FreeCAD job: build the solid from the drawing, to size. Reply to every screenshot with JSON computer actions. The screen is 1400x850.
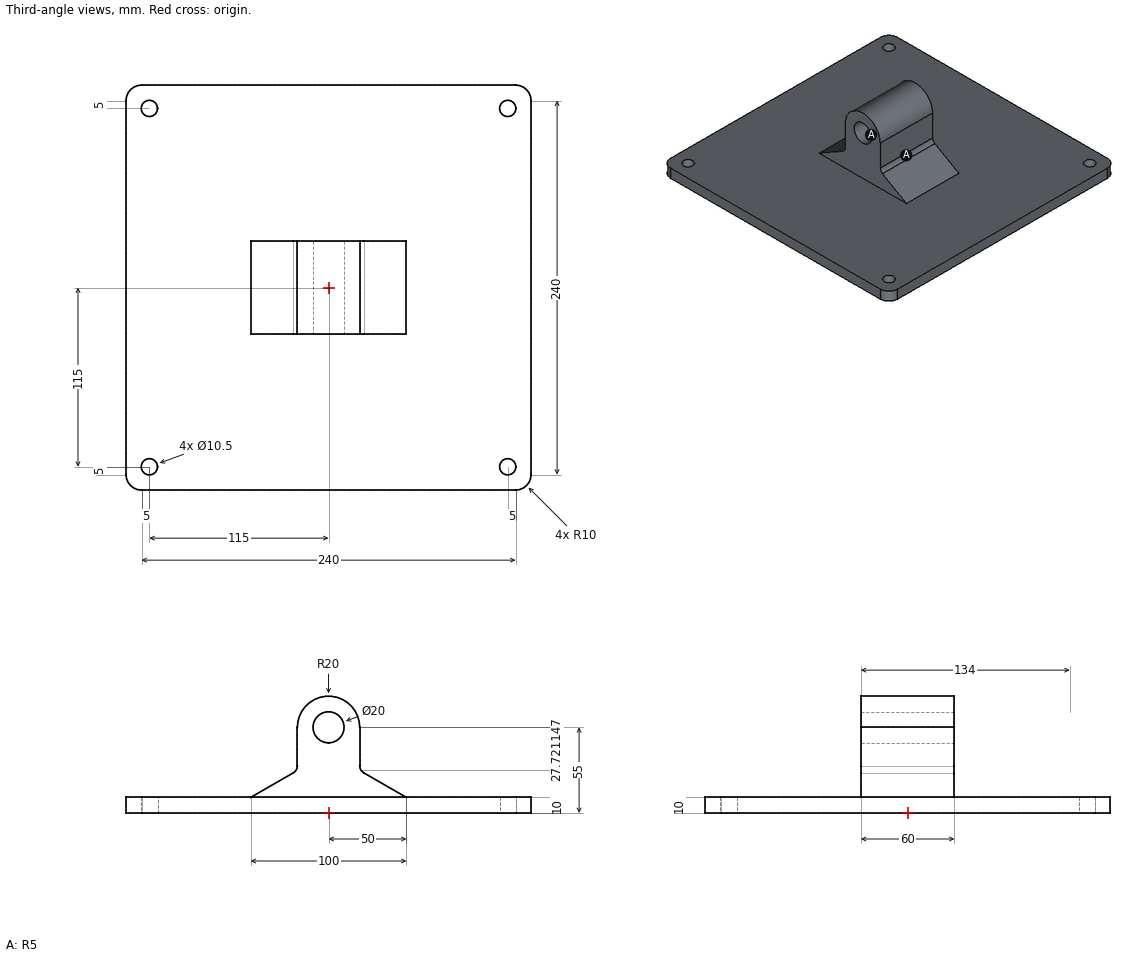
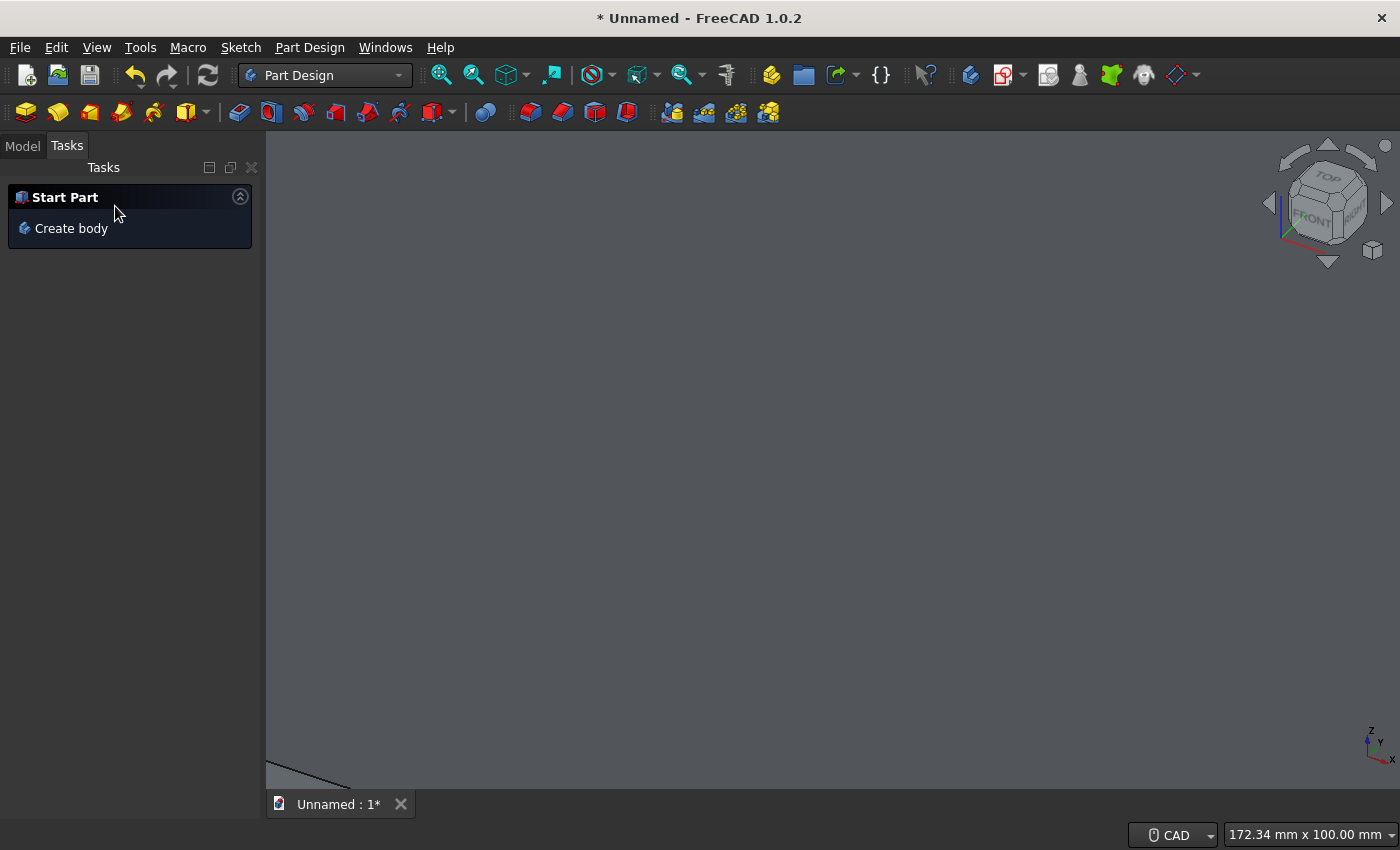
{"action": "left_click", "coordinate": [442, 76]}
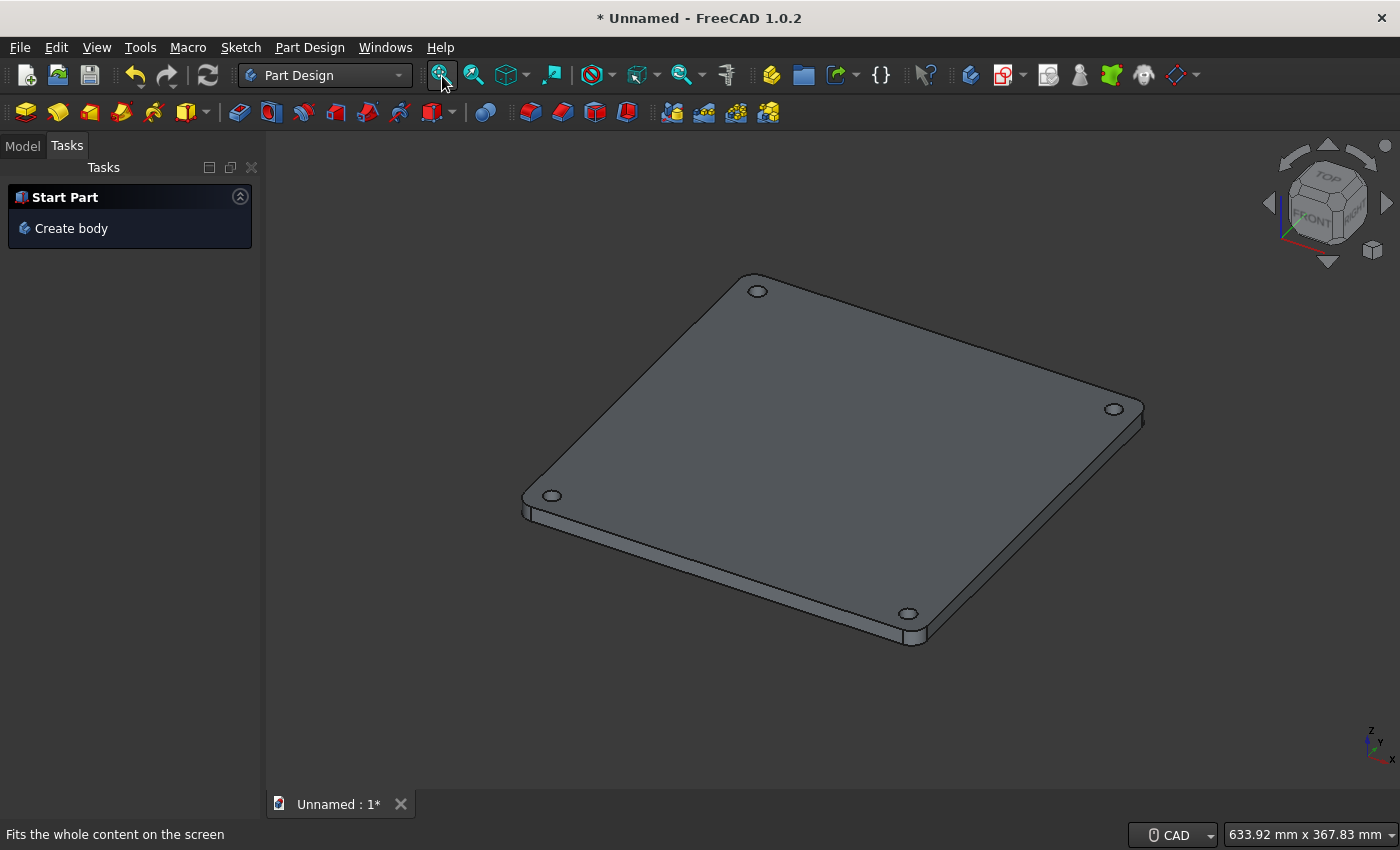
{"action": "left_click", "coordinate": [1004, 76]}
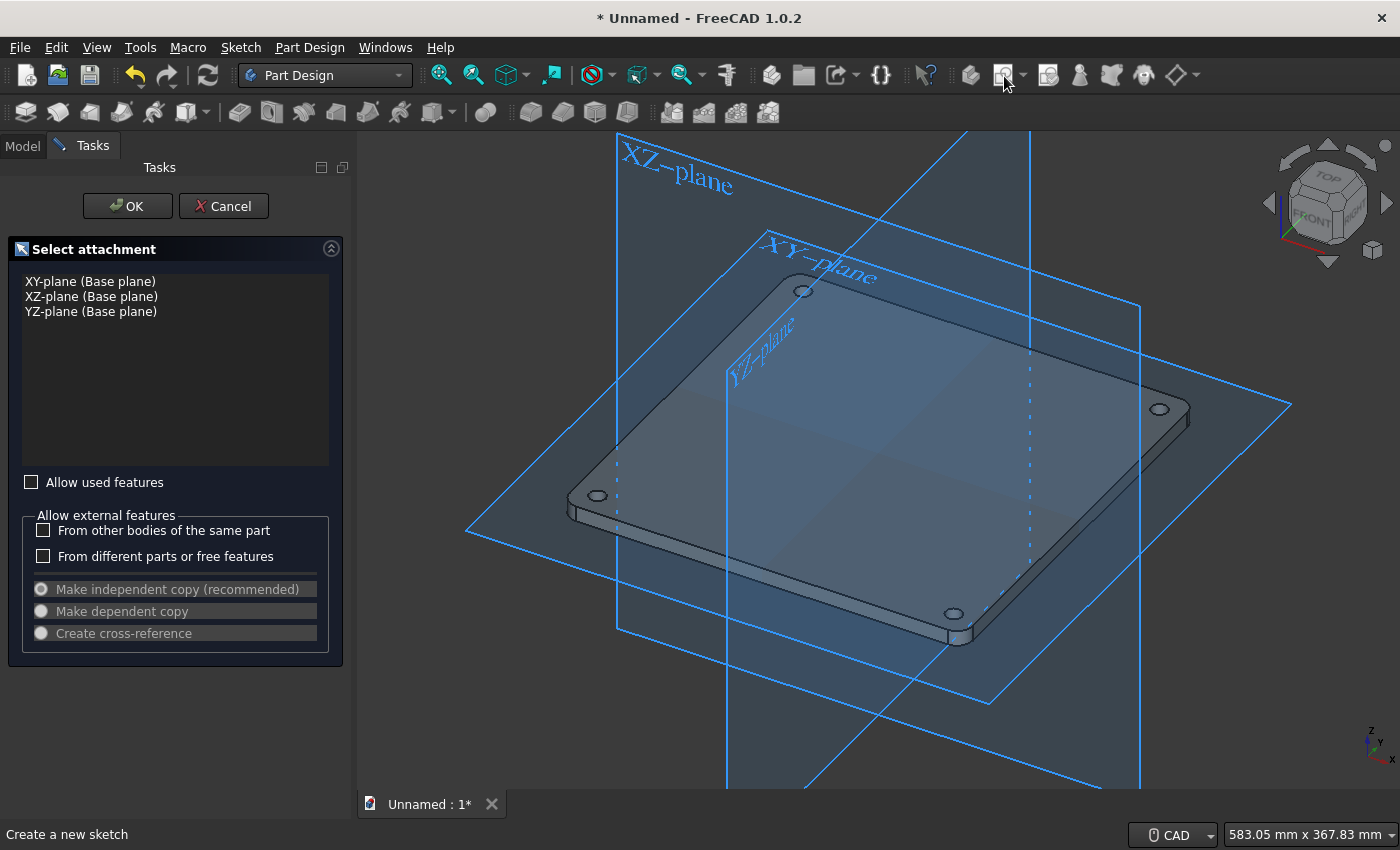
{"action": "left_click", "coordinate": [82, 296]}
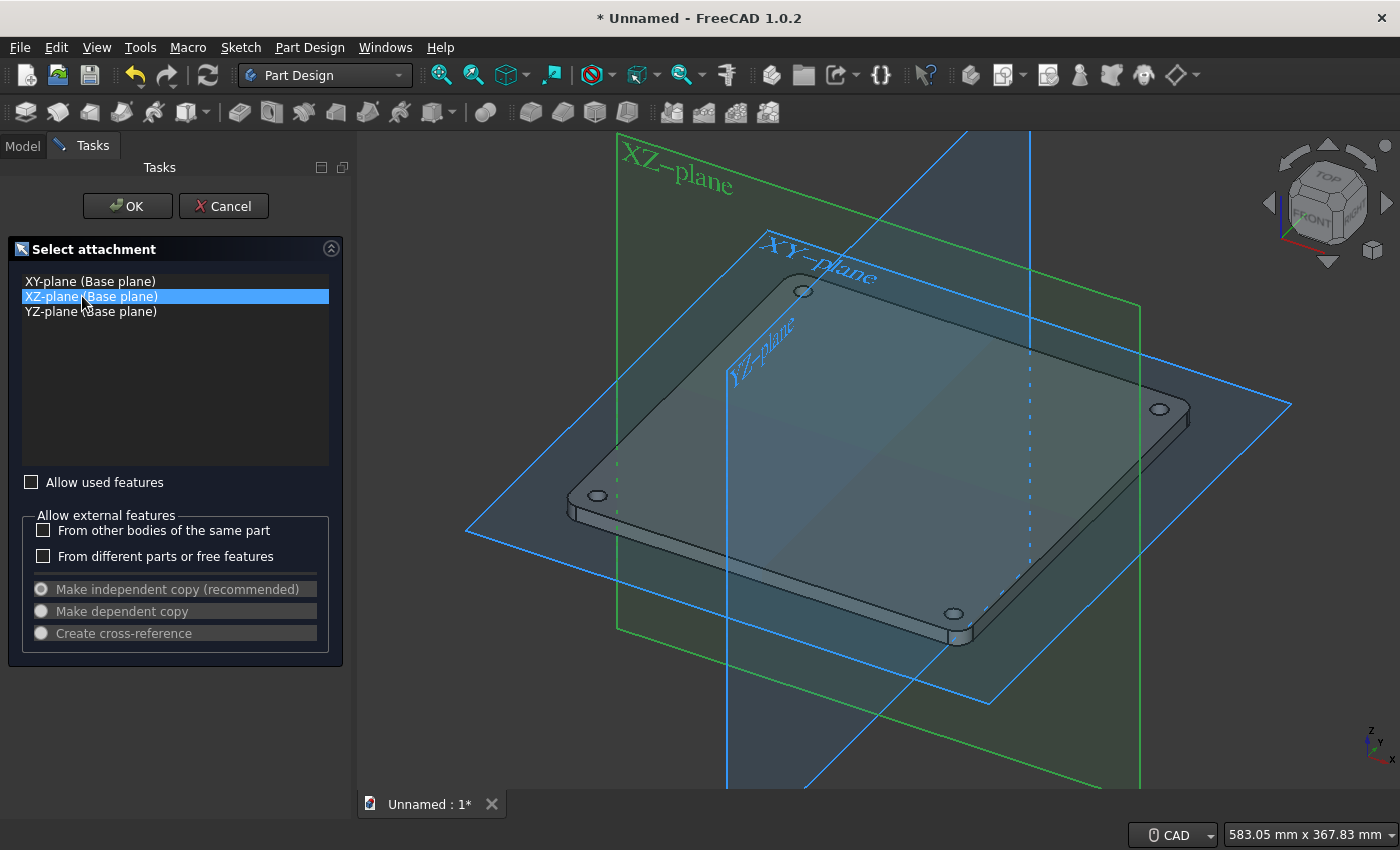
{"action": "left_click", "coordinate": [128, 206]}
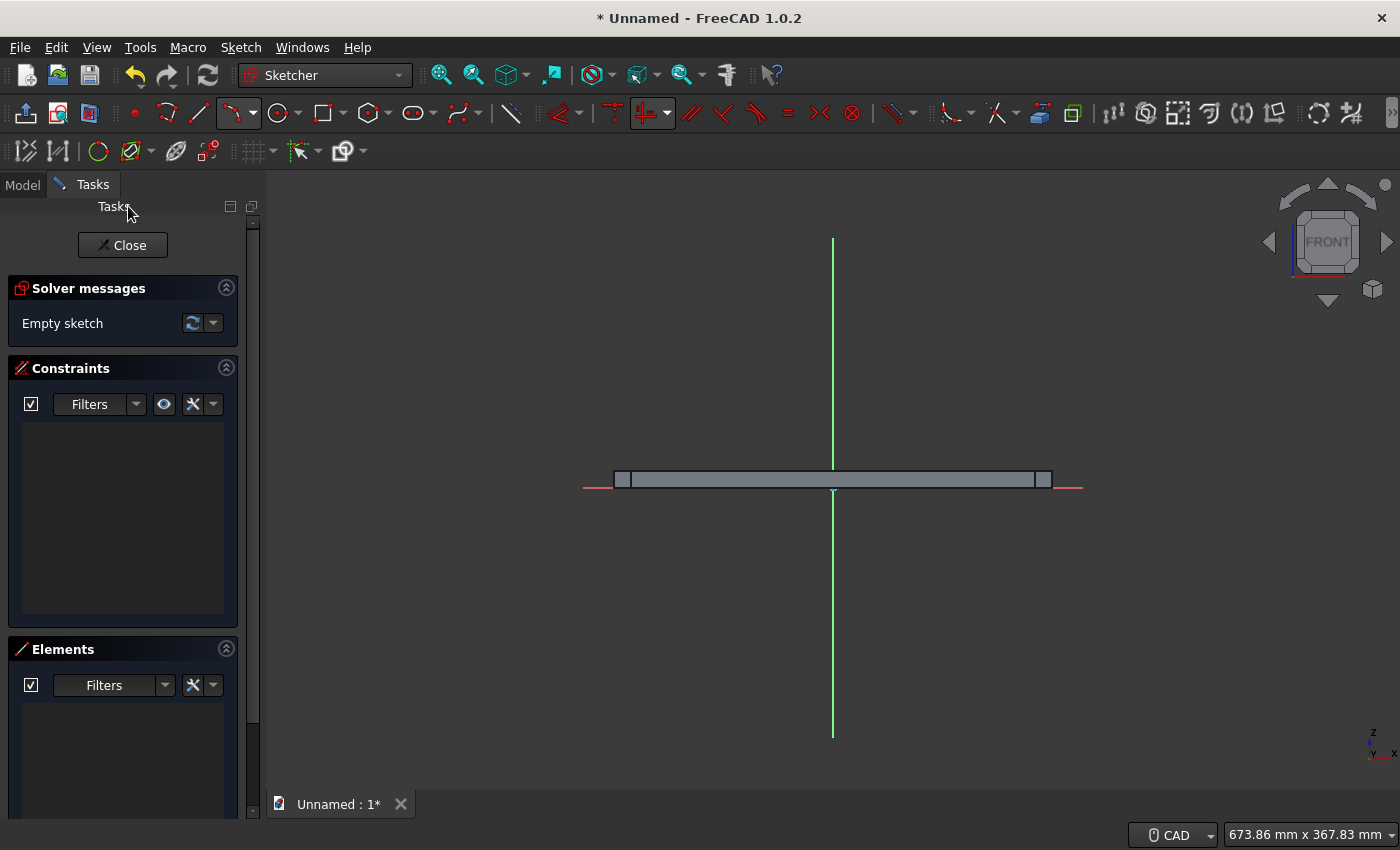
{"action": "left_click", "coordinate": [90, 114]}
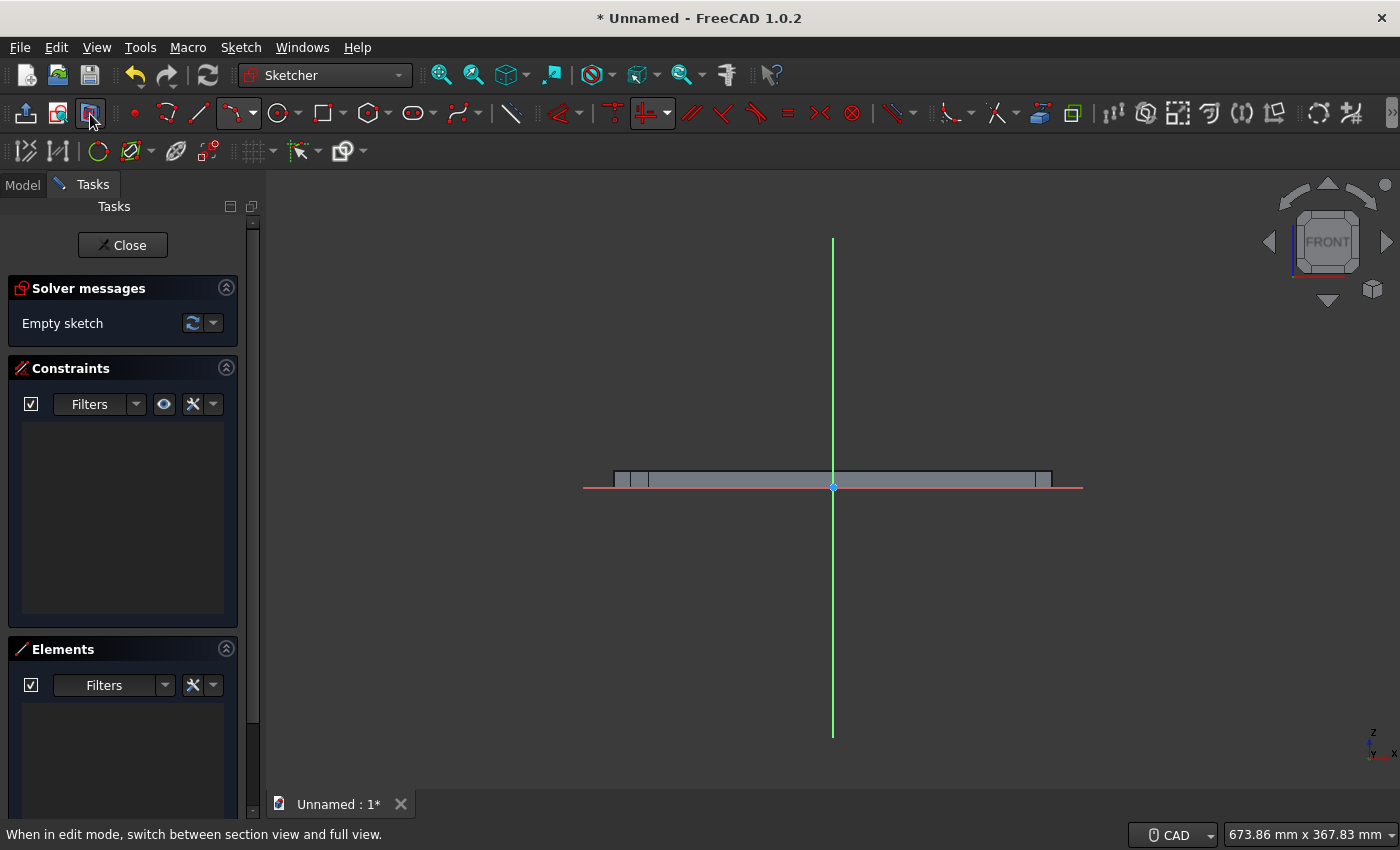
{"action": "scroll", "coordinate": [863, 401], "scroll_direction": "up", "scroll_amount": 6}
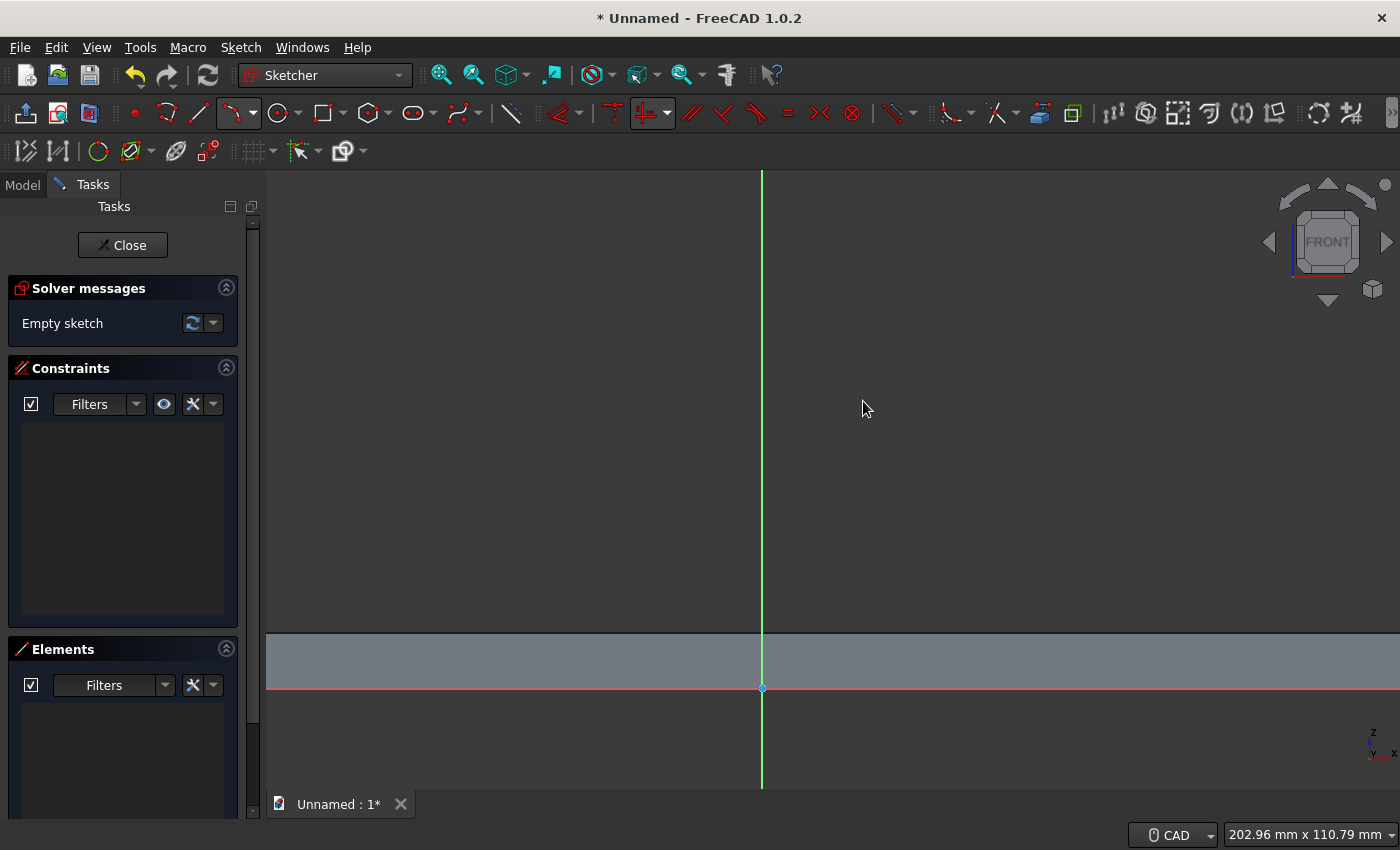
{"action": "left_click", "coordinate": [168, 114]}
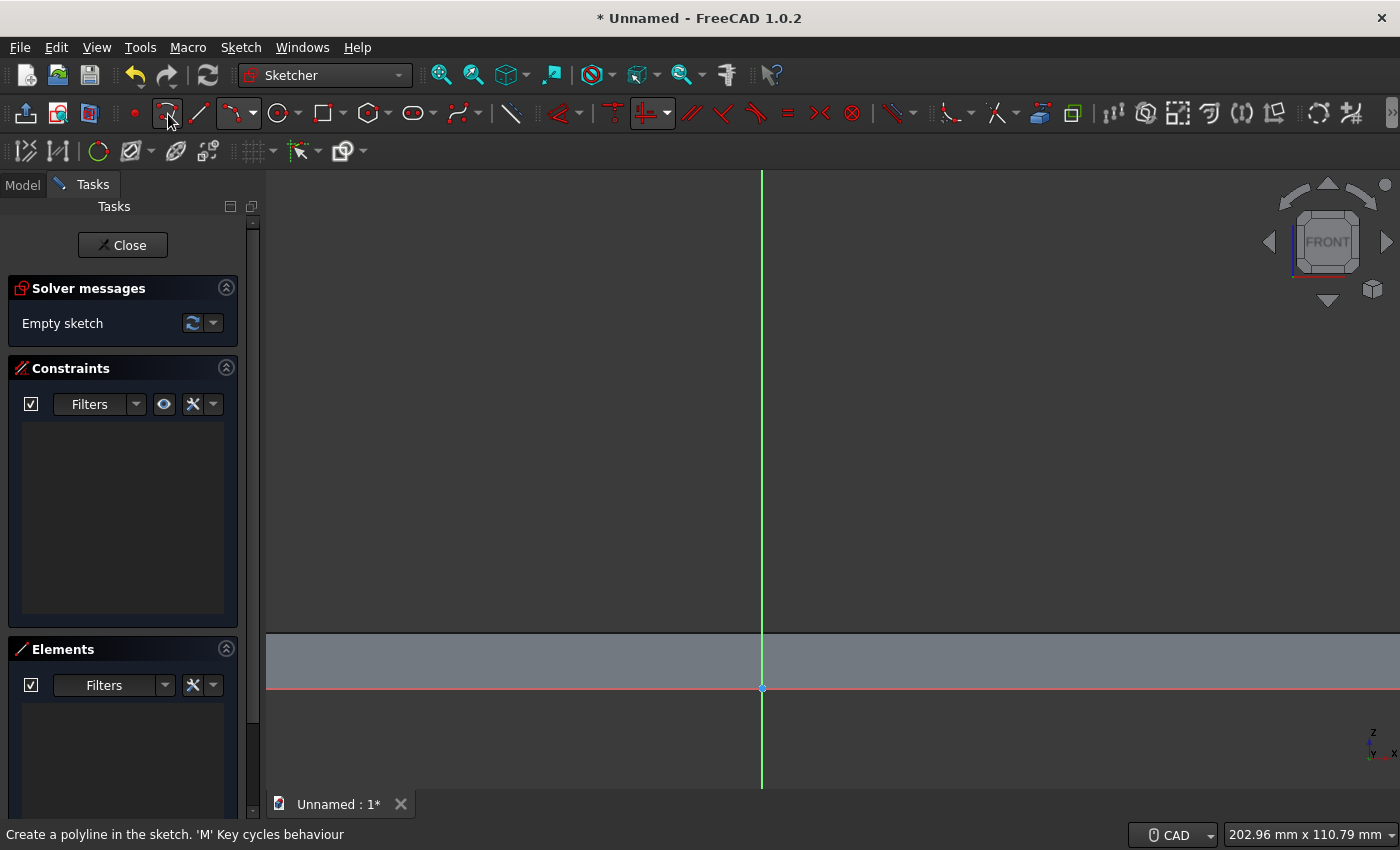
{"action": "left_click", "coordinate": [874, 381]}
{"action": "left_click", "coordinate": [874, 536]}
{"action": "left_click", "coordinate": [1042, 633]}
{"action": "left_click", "coordinate": [483, 633]}
{"action": "left_click", "coordinate": [650, 536]}
{"action": "left_click", "coordinate": [650, 381]}
{"action": "right_click", "coordinate": [650, 381]}